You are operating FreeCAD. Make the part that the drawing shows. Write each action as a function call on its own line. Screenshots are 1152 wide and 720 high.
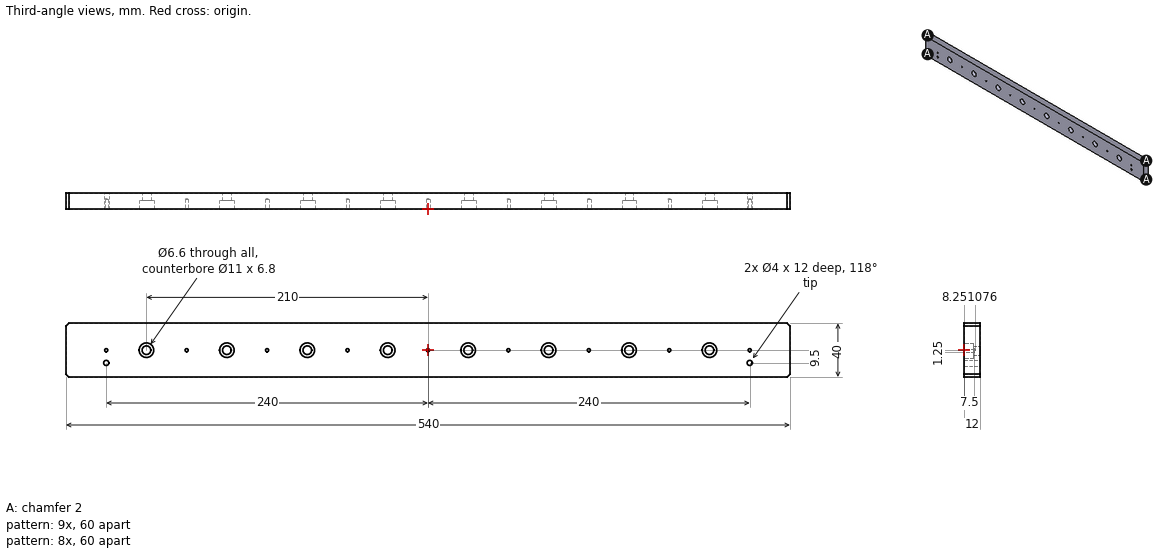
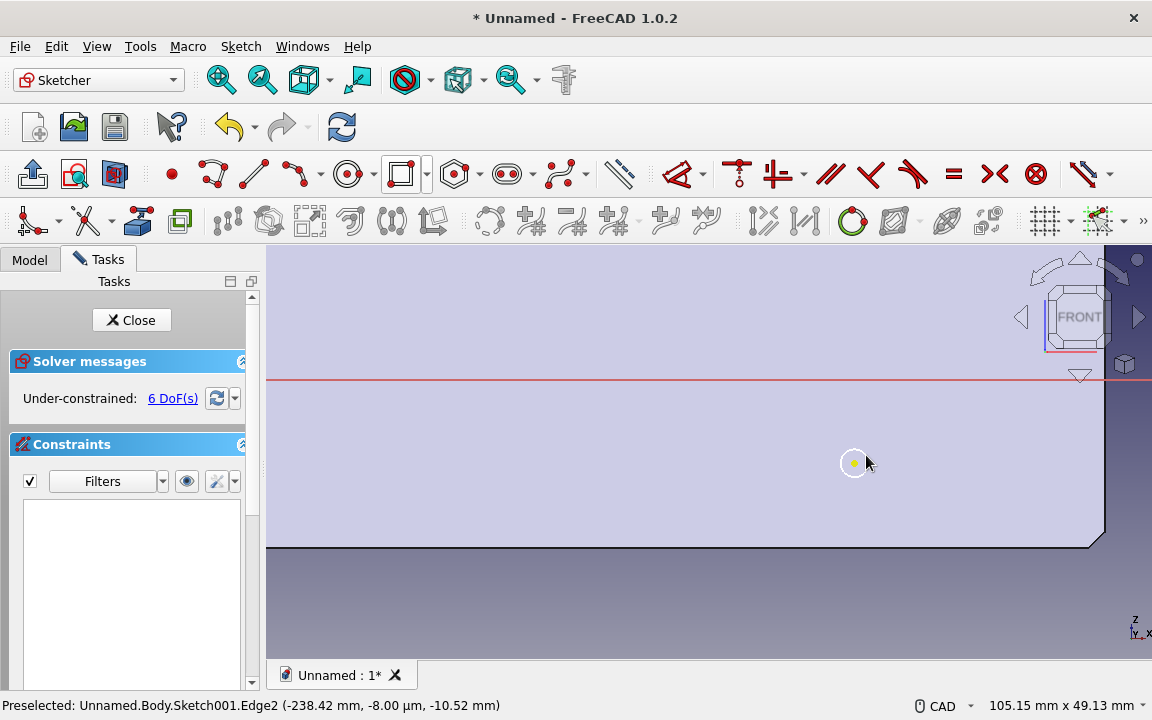
click(864, 453)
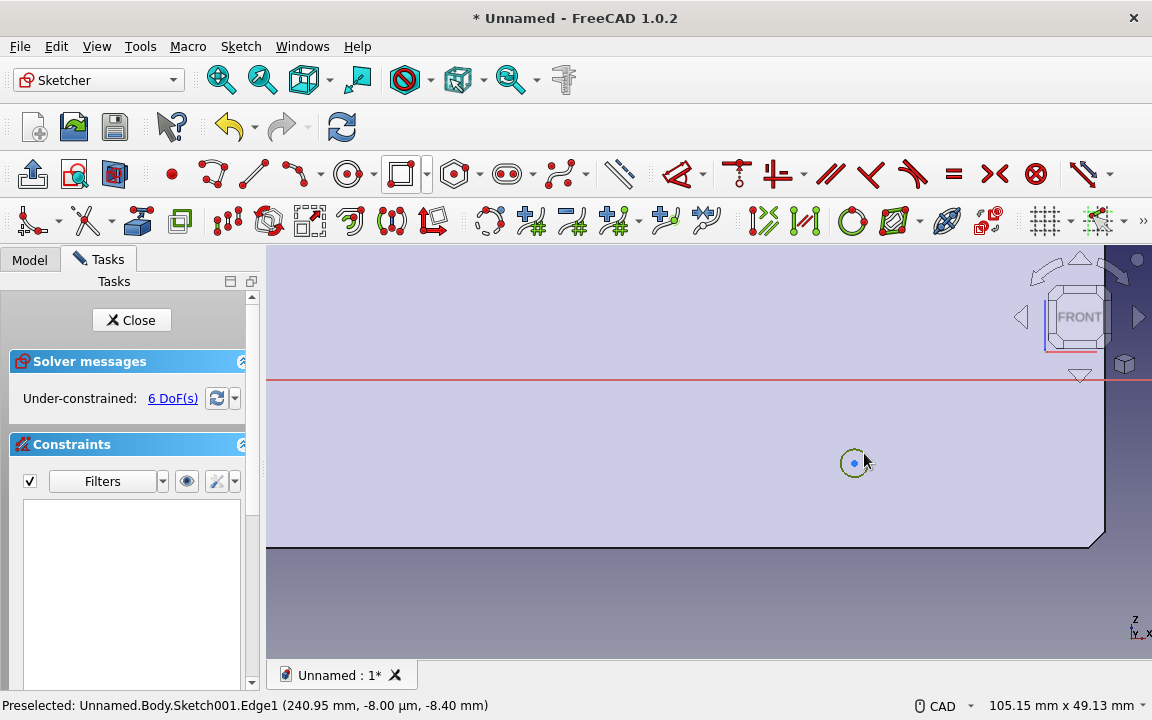
scroll(866, 455, down, 11)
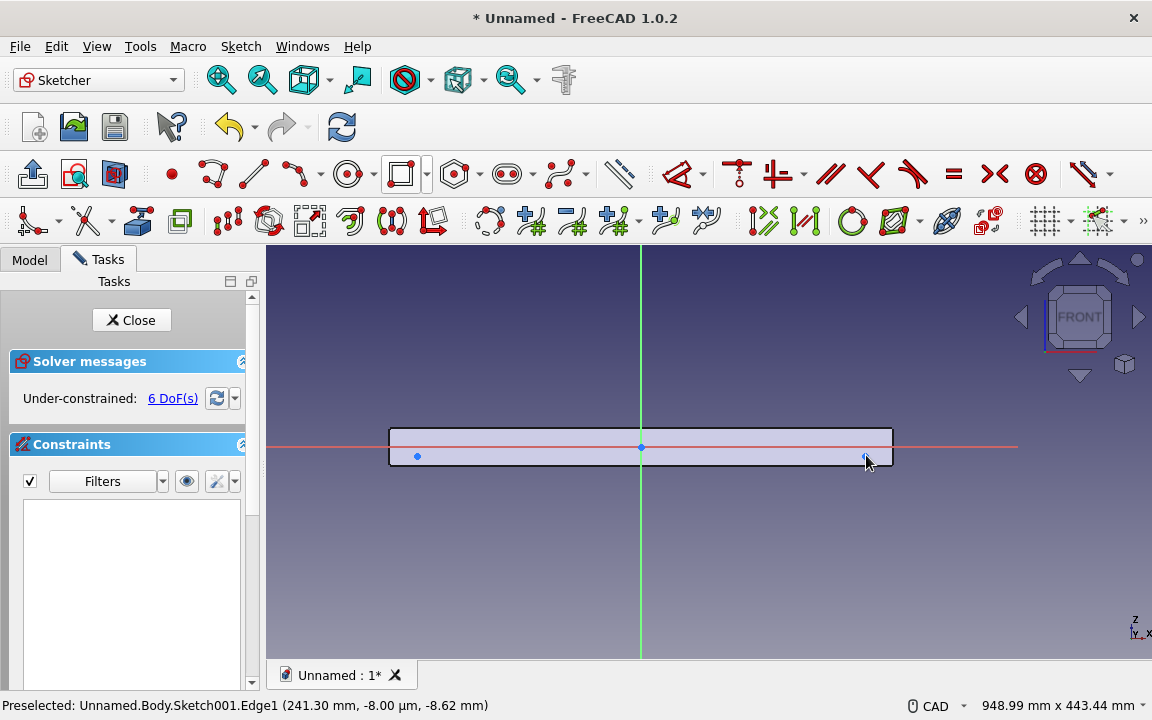
scroll(418, 456, up, 12)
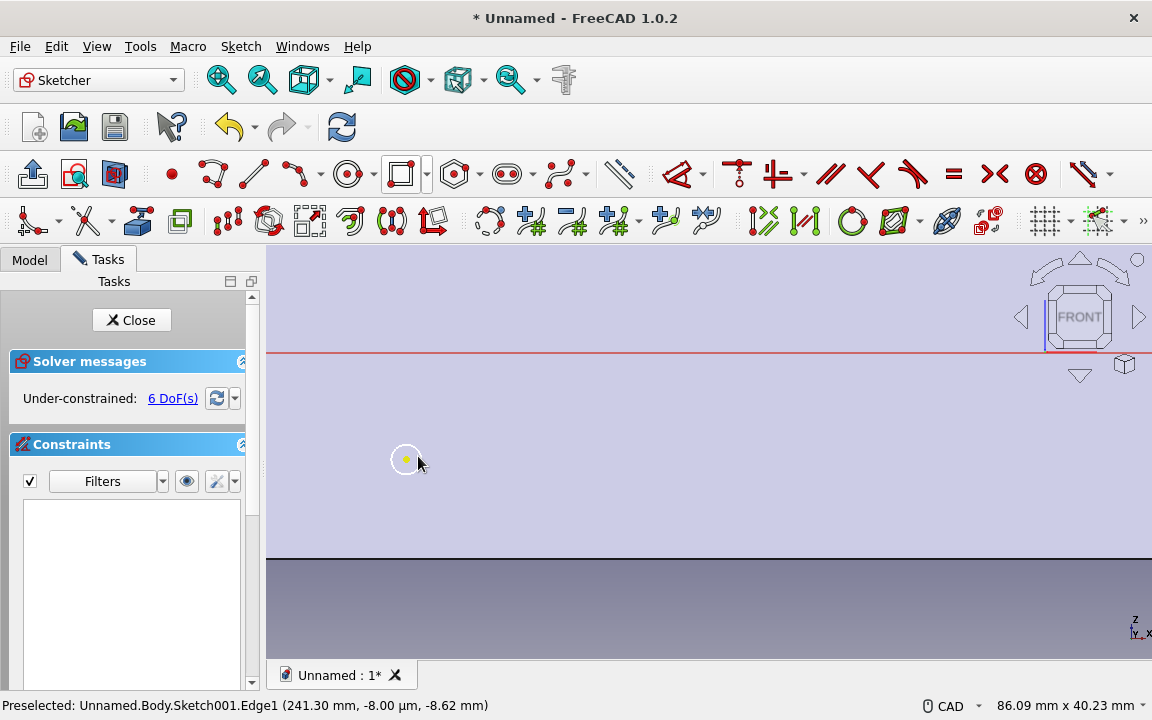
click(417, 449)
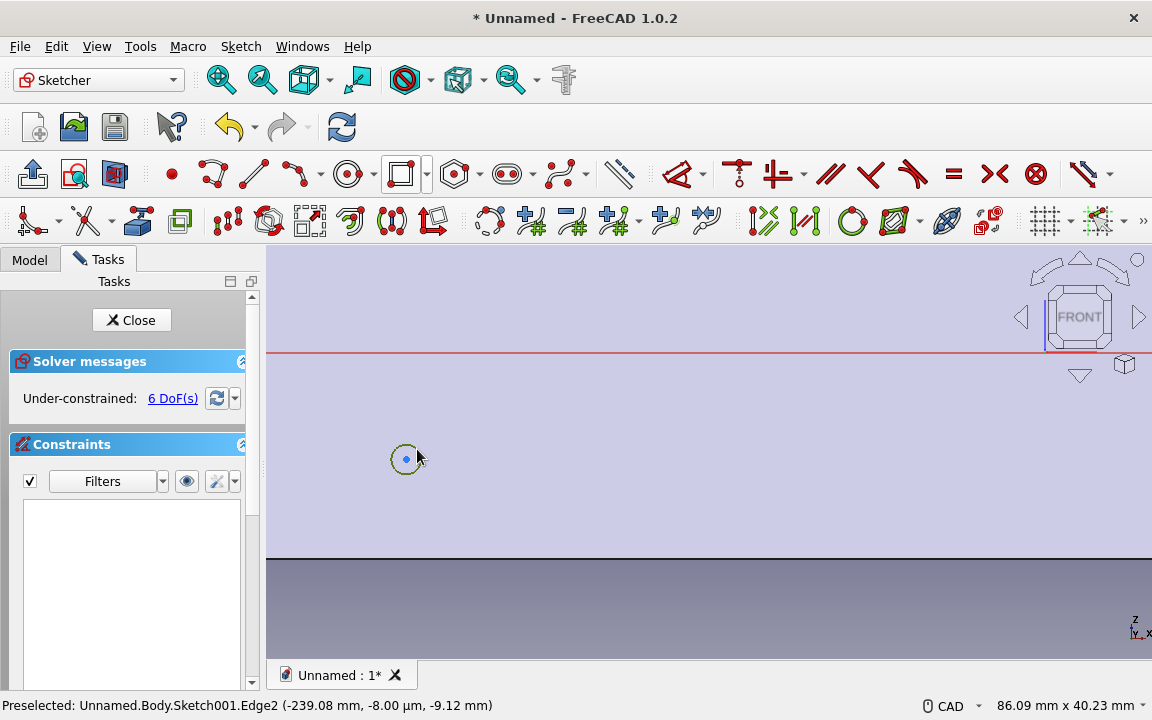
click(954, 174)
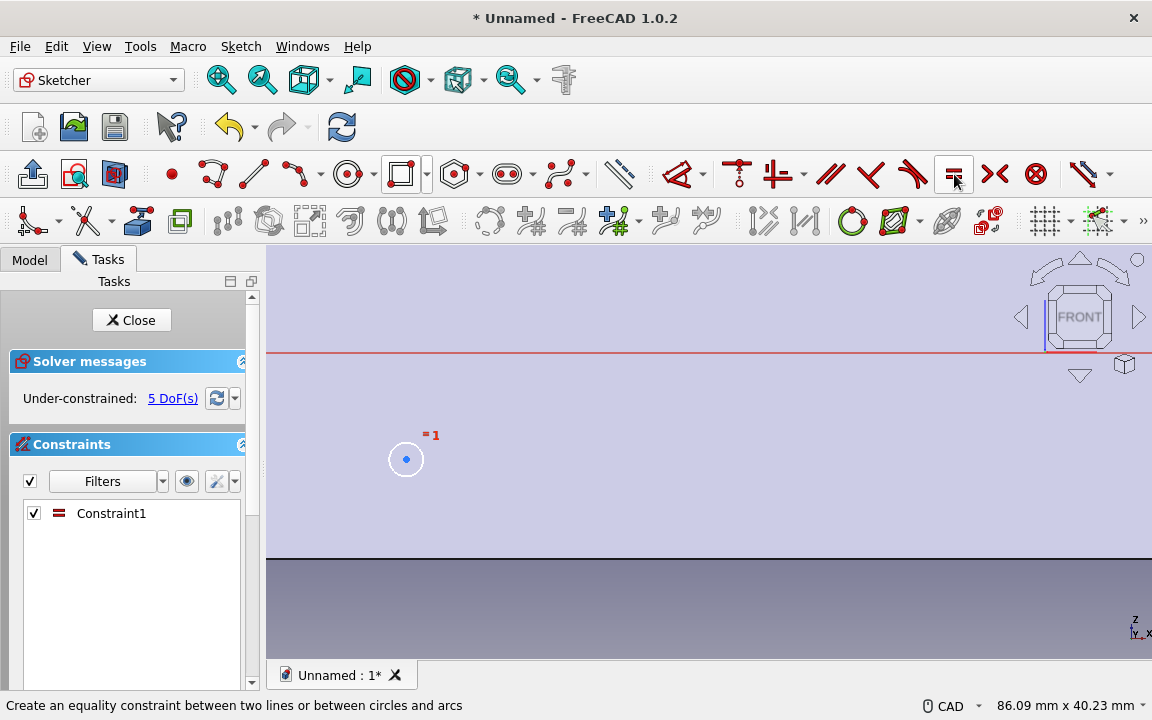
scroll(418, 456, down, 12)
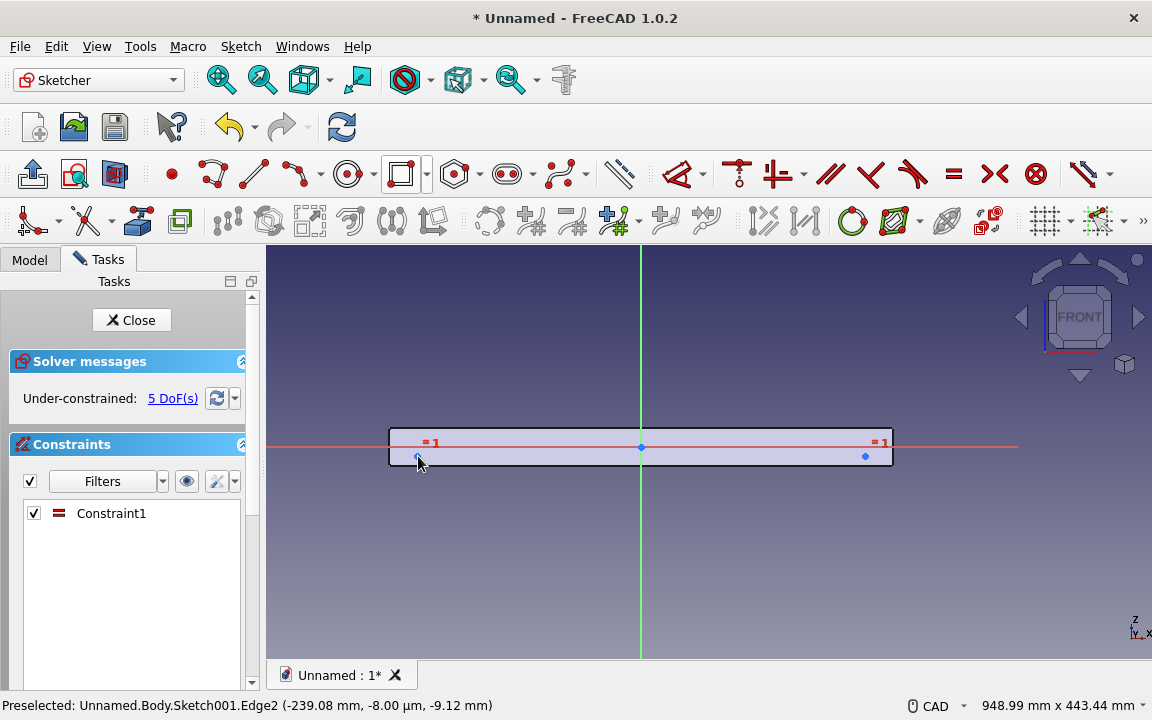
click(865, 456)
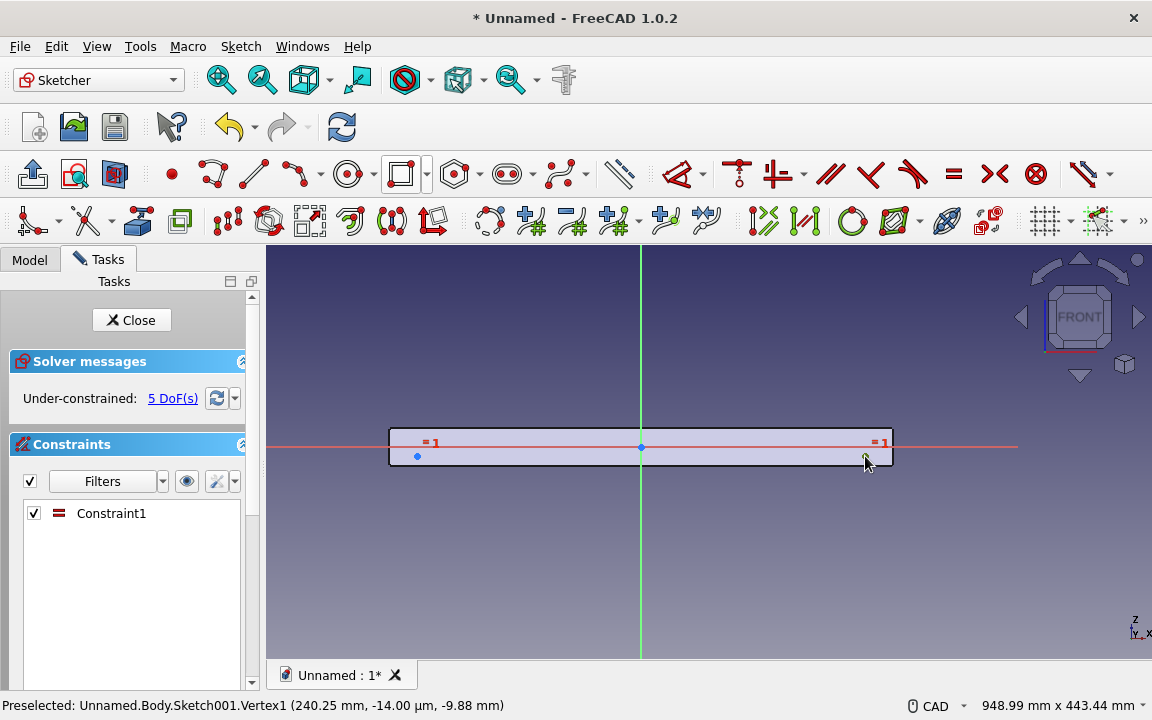
click(417, 457)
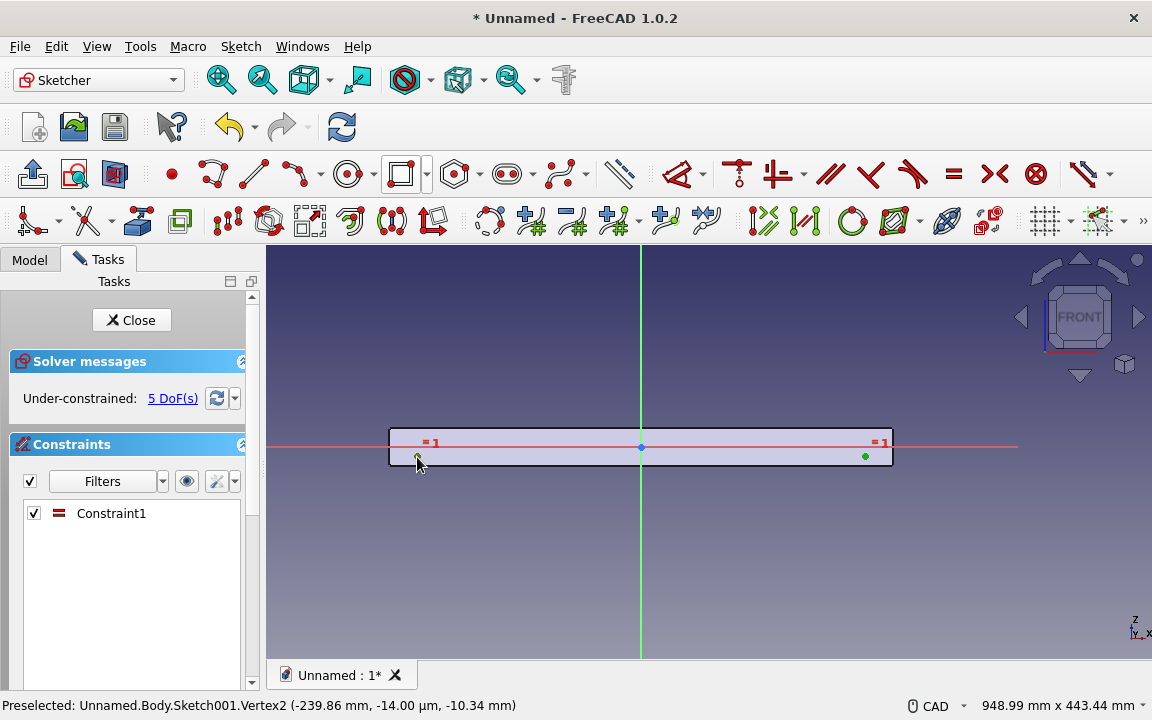
click(804, 174)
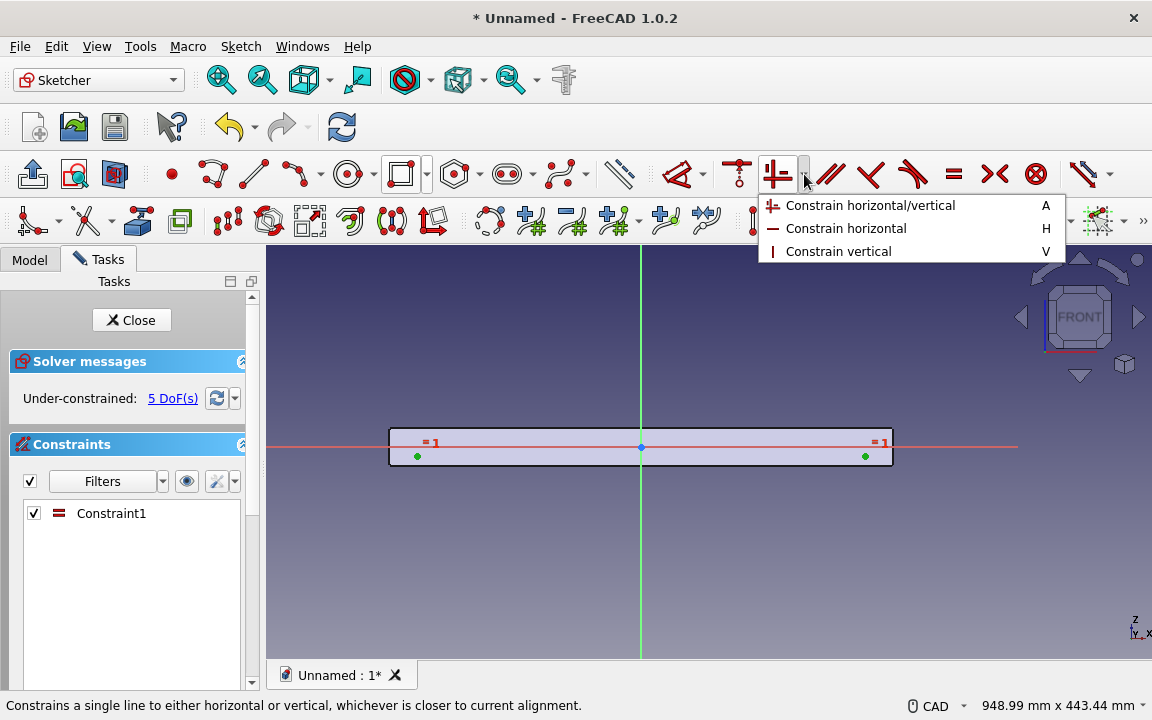
click(912, 228)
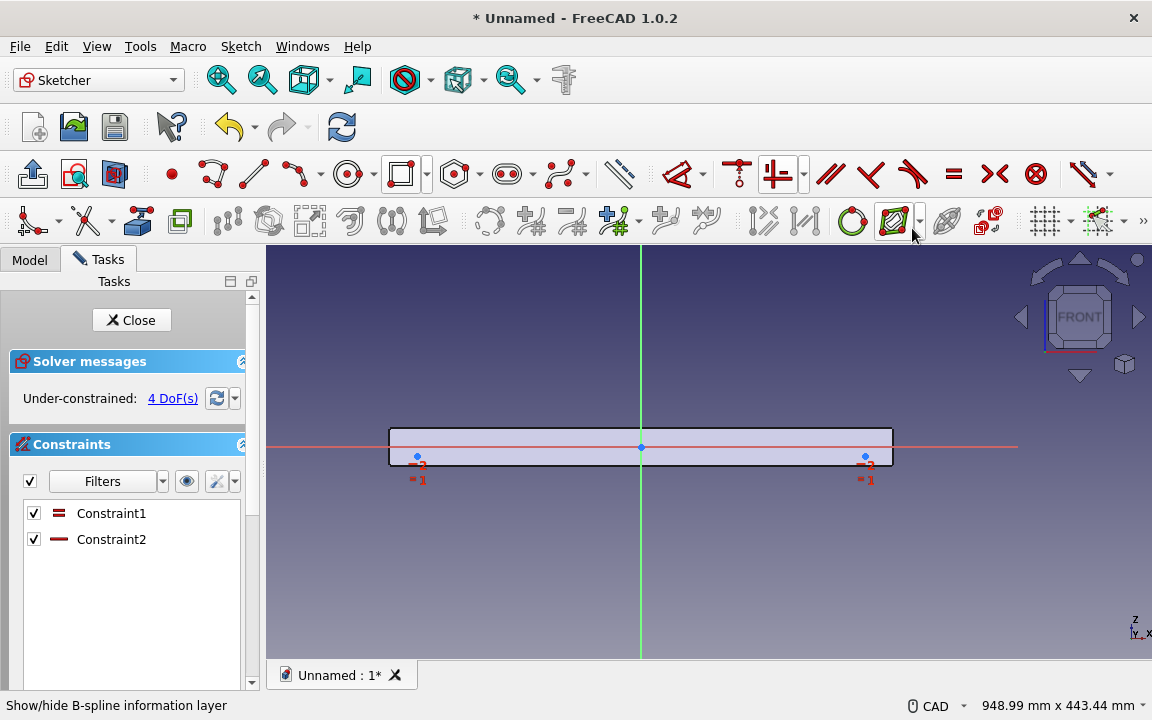
key(d)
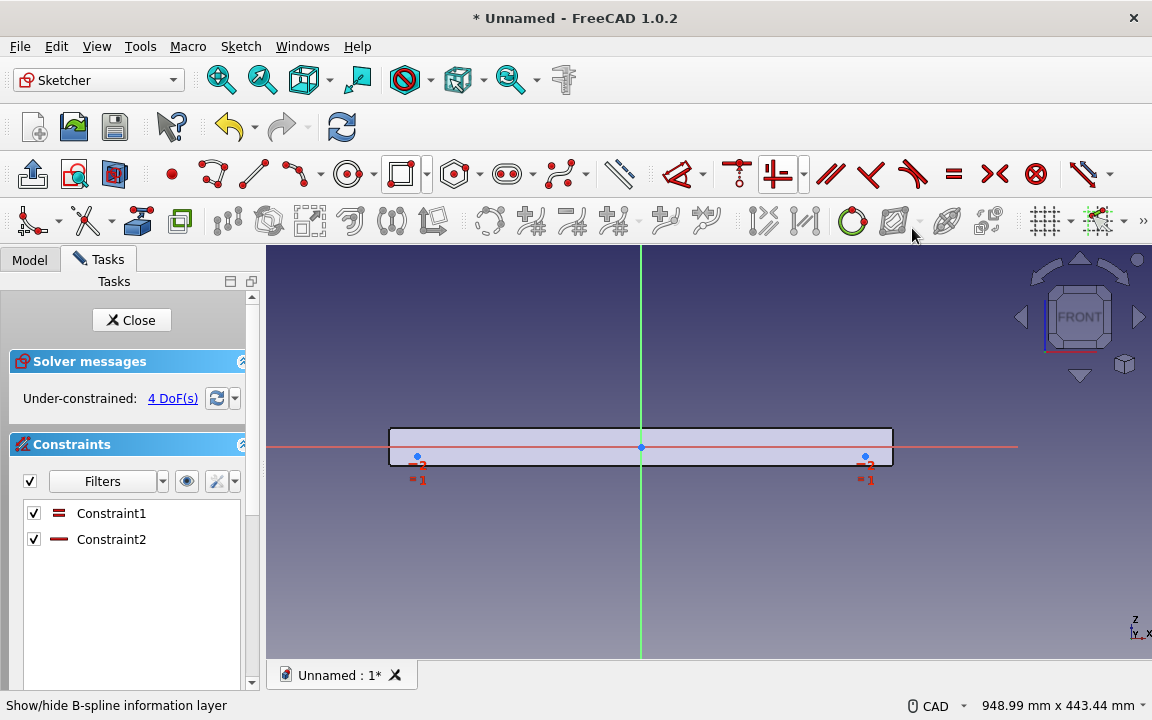
scroll(864, 456, up, 12)